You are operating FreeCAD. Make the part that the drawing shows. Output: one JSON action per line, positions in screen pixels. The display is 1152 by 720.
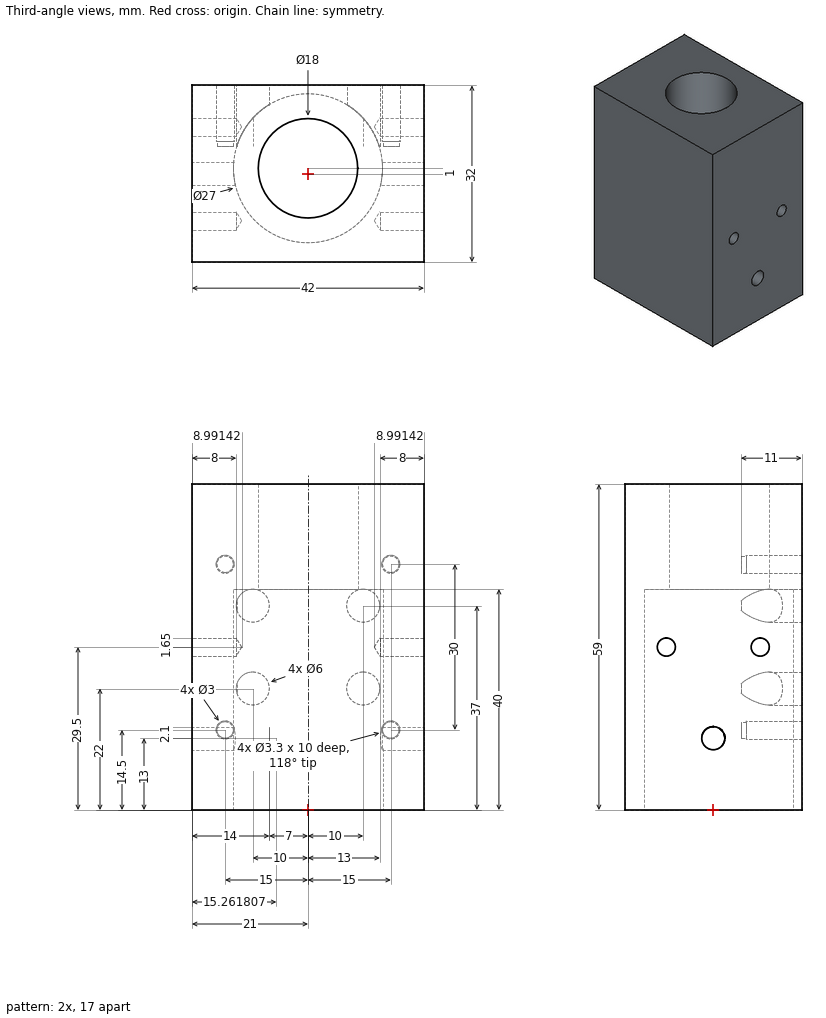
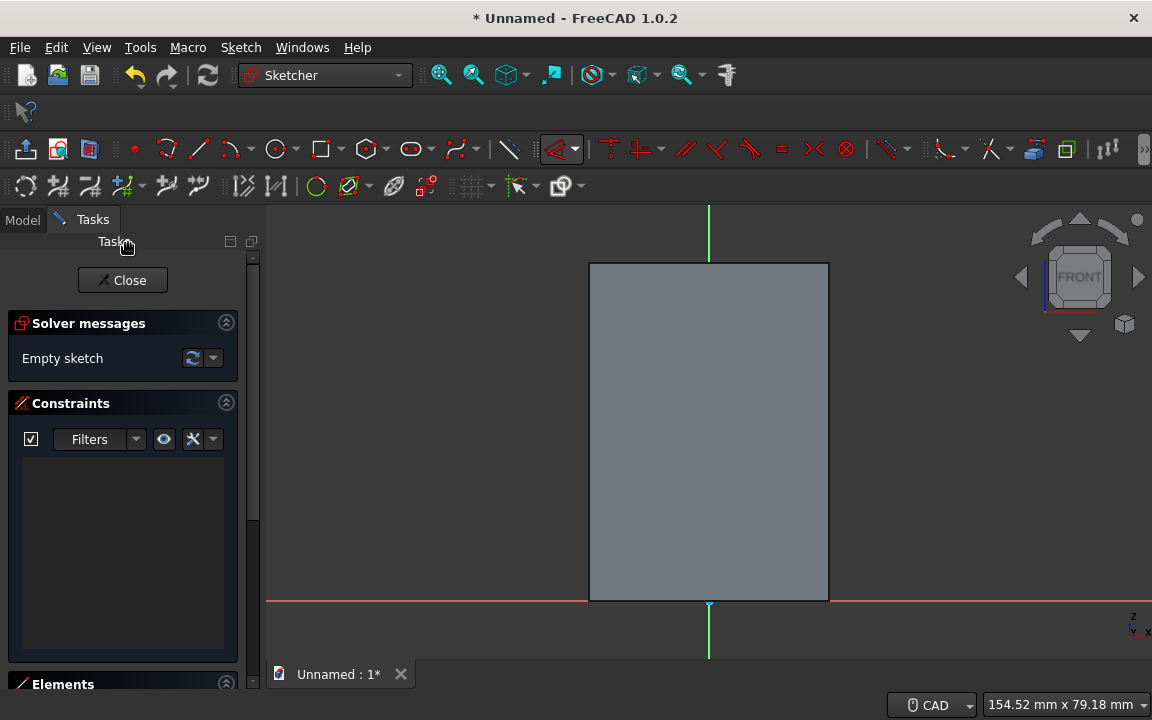
{"action": "key", "text": "q s"}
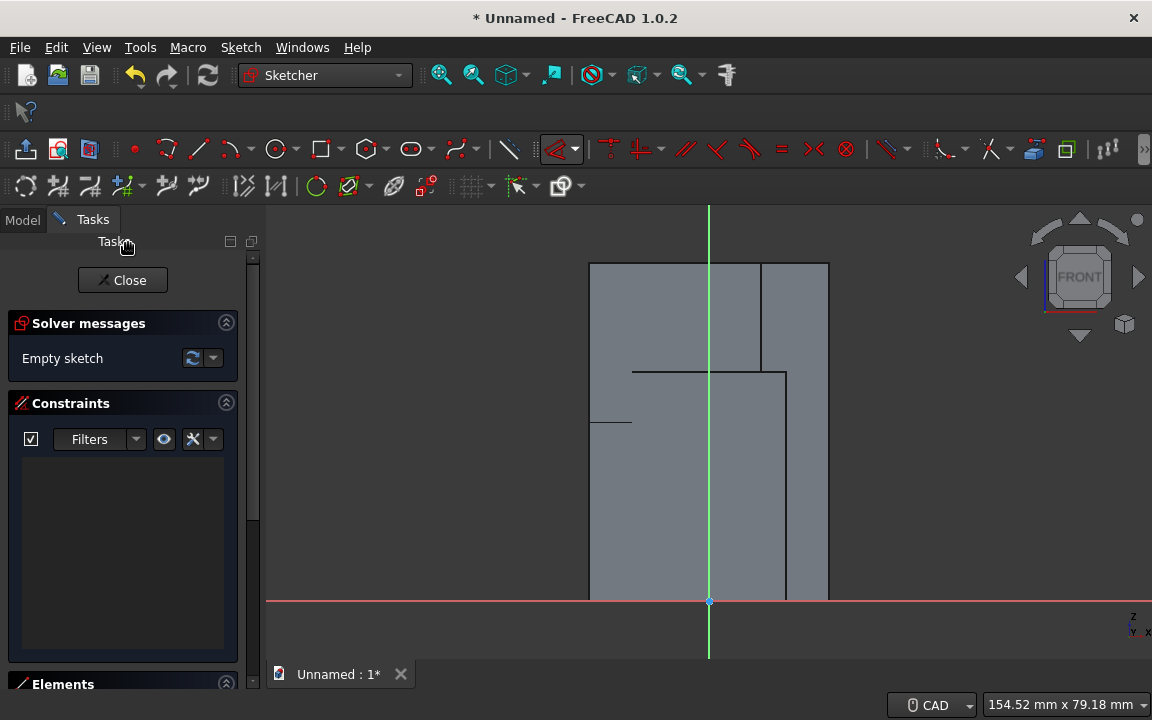
{"action": "scroll", "coordinate": [654, 612], "scroll_direction": "up", "scroll_amount": 6}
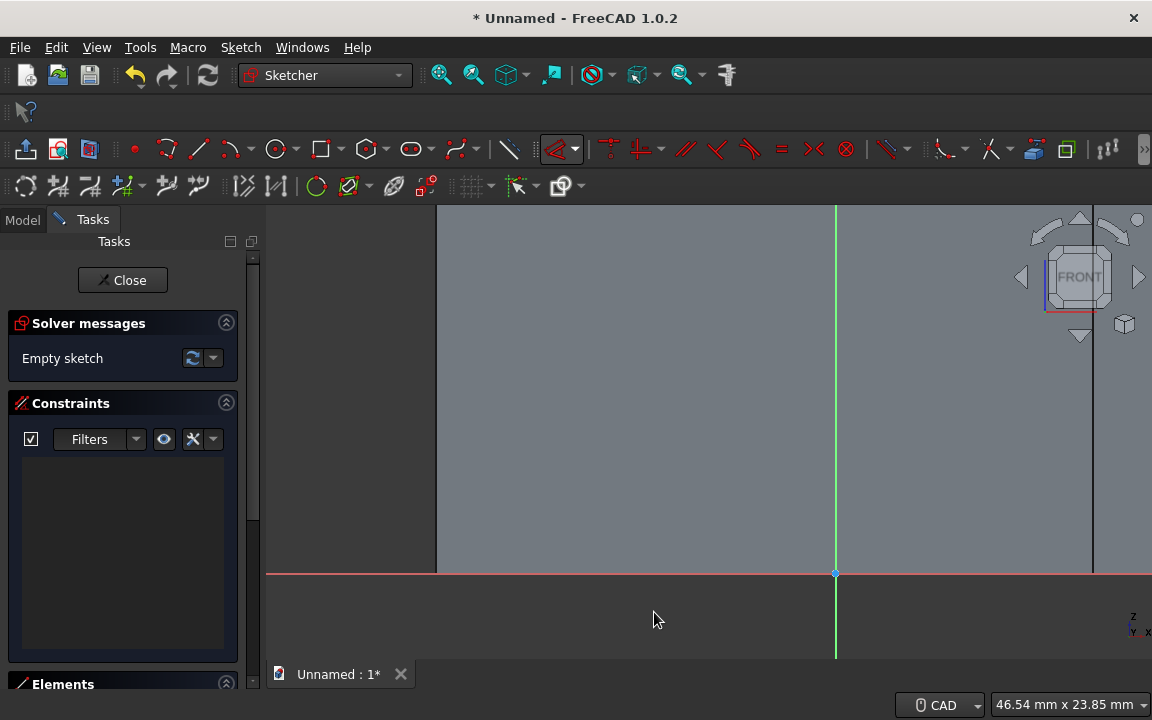
{"action": "left_click", "coordinate": [168, 150]}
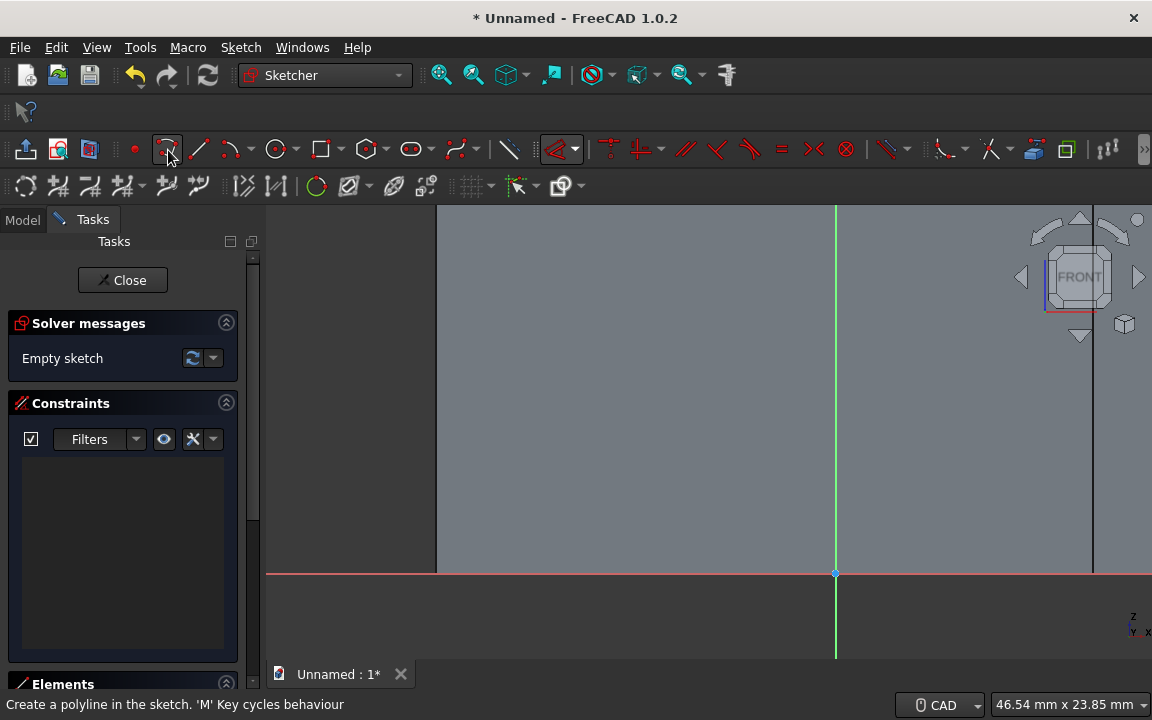
{"action": "left_click", "coordinate": [726, 326]}
{"action": "left_click", "coordinate": [436, 326]}
{"action": "left_click", "coordinate": [436, 286]}
{"action": "left_click", "coordinate": [702, 286]}
{"action": "left_click", "coordinate": [726, 327]}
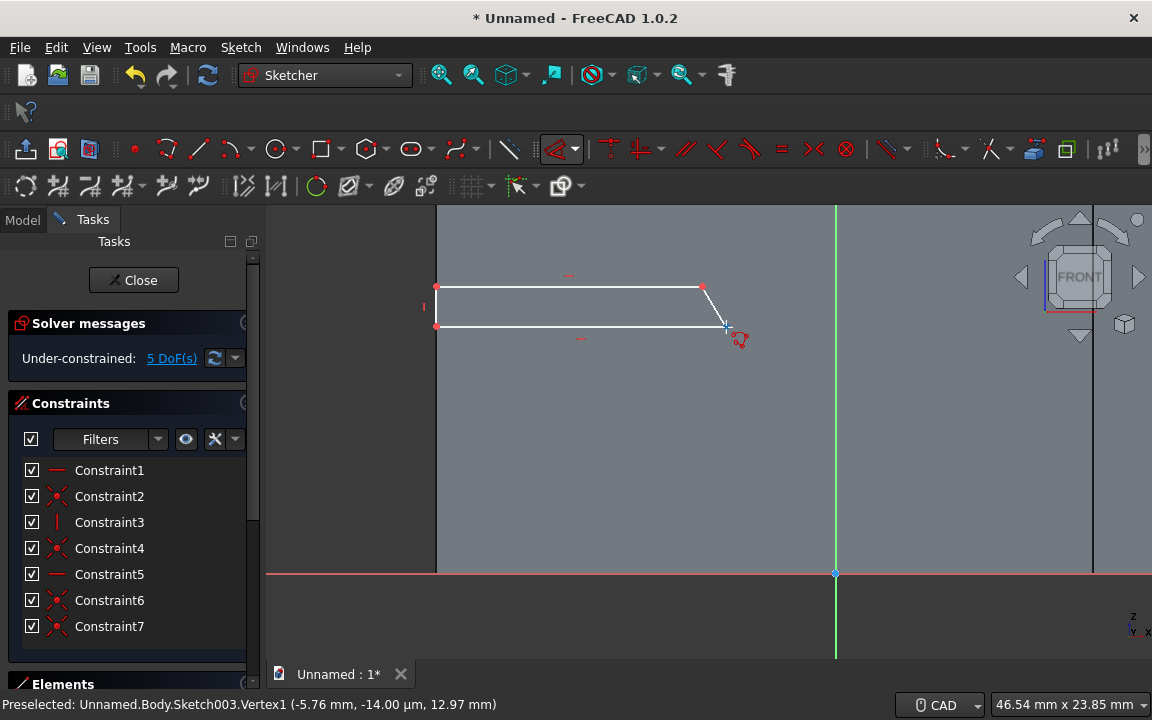
{"action": "key", "text": "g l"}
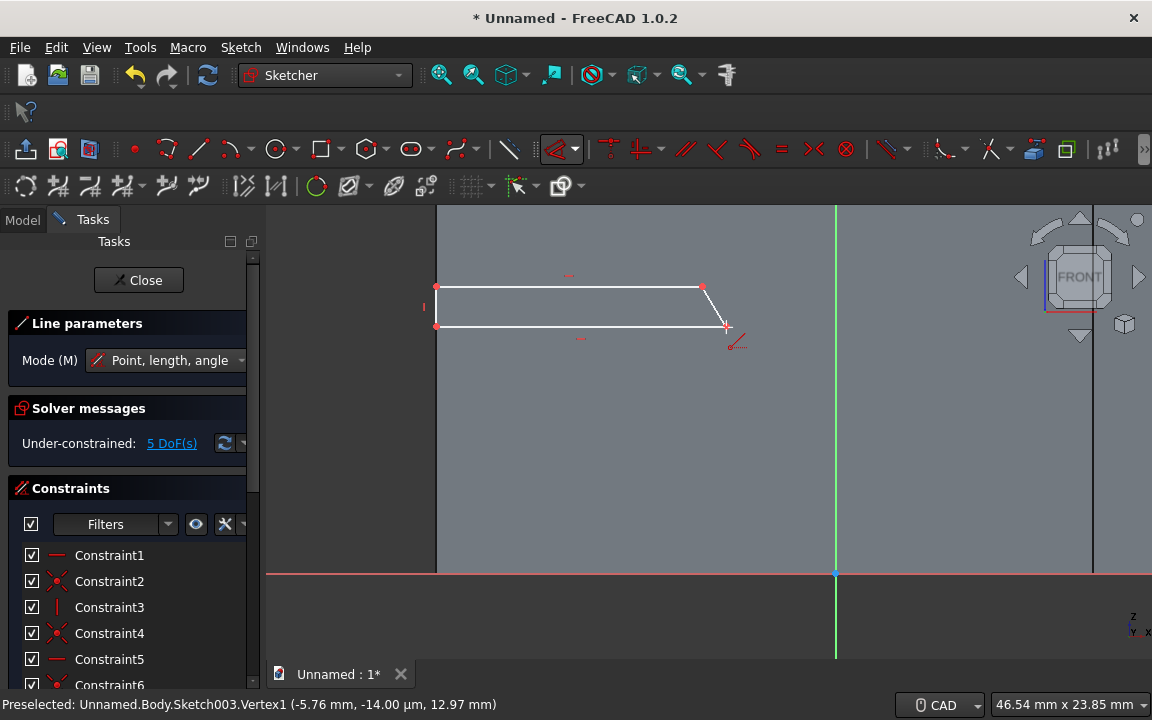
{"action": "left_click", "coordinate": [755, 326]}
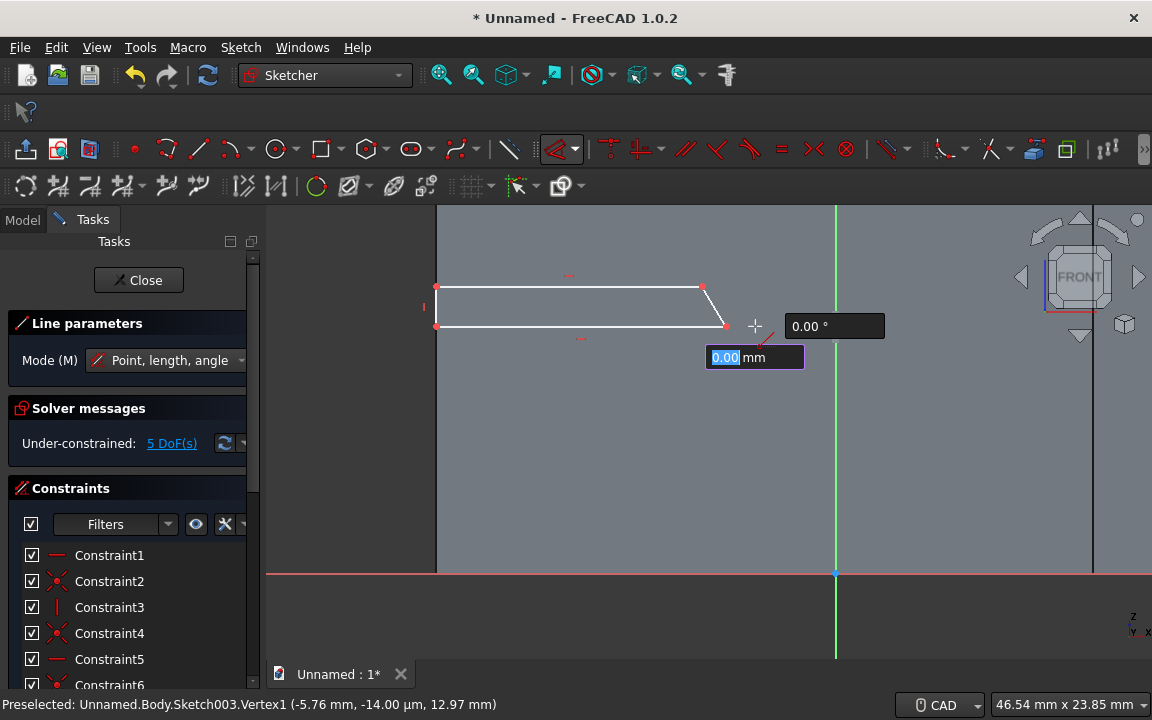
{"action": "scroll", "coordinate": [843, 326], "scroll_direction": "up", "scroll_amount": 5}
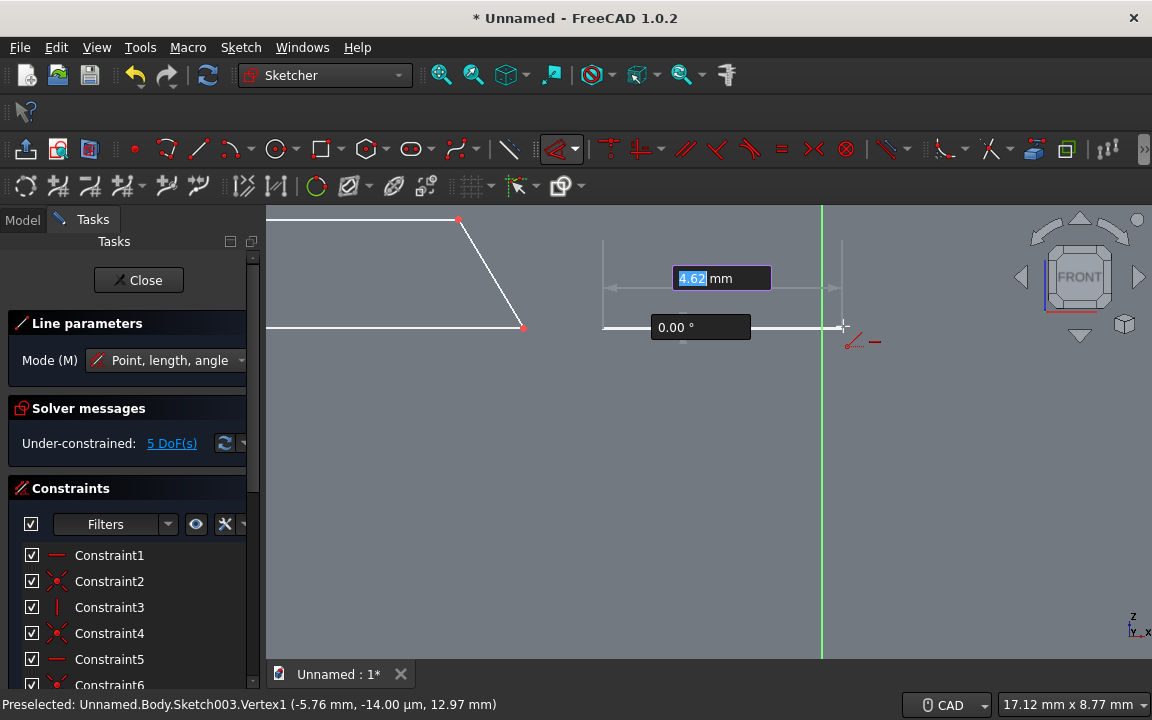
{"action": "left_click", "coordinate": [841, 326]}
{"action": "key", "text": "Escape"}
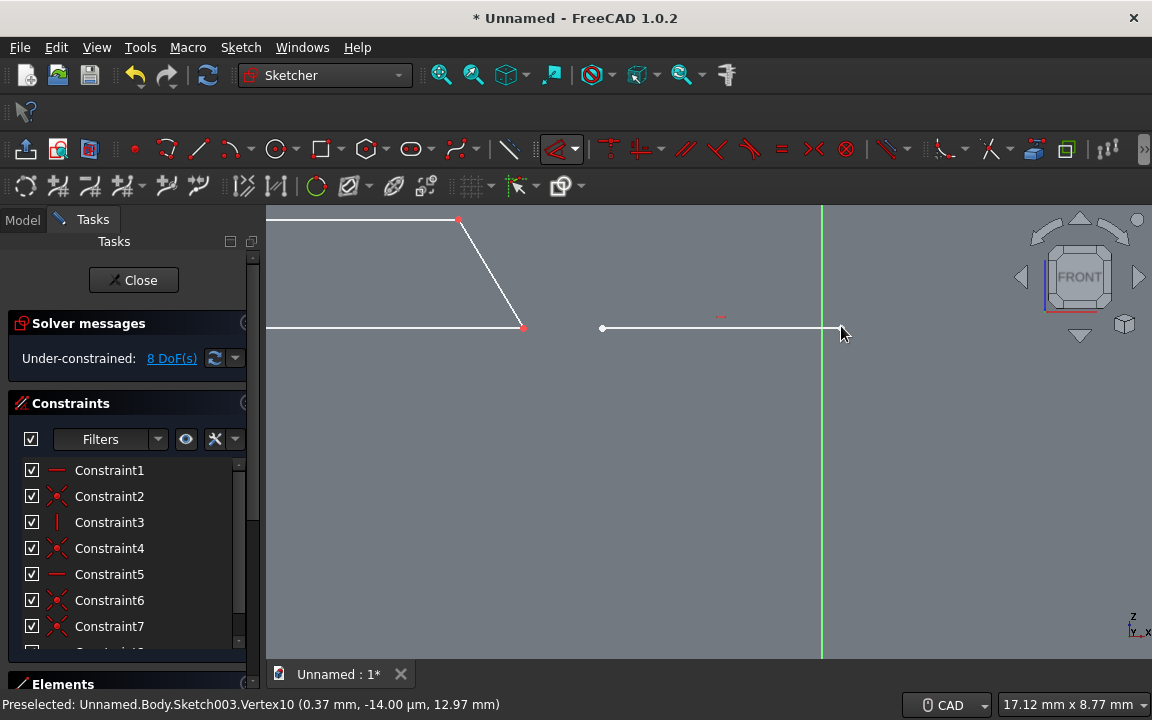
{"action": "left_click", "coordinate": [674, 328]}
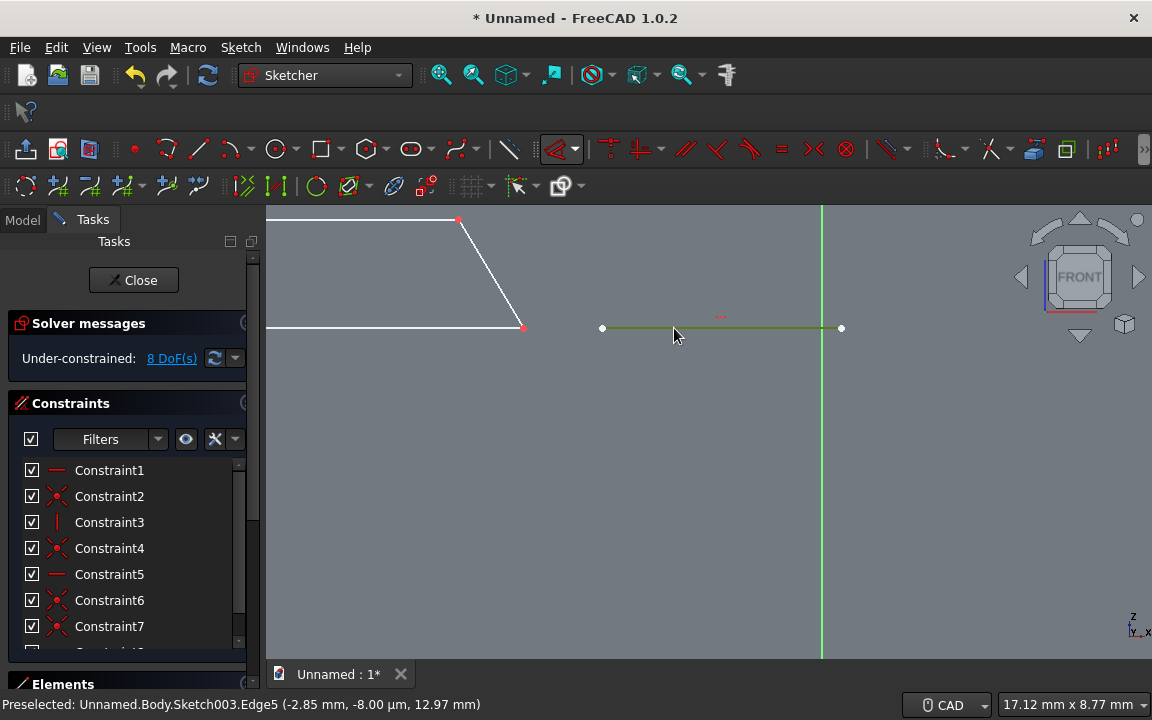
{"action": "left_click", "coordinate": [510, 150]}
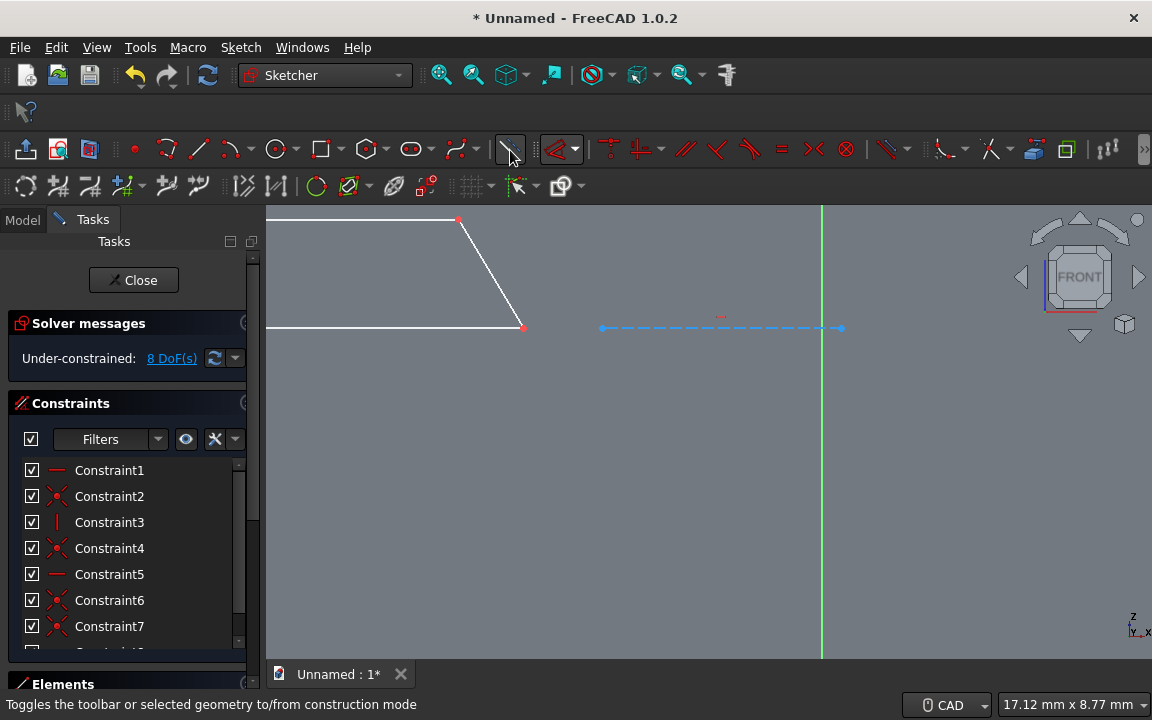
{"action": "scroll", "coordinate": [846, 329], "scroll_direction": "down", "scroll_amount": 5}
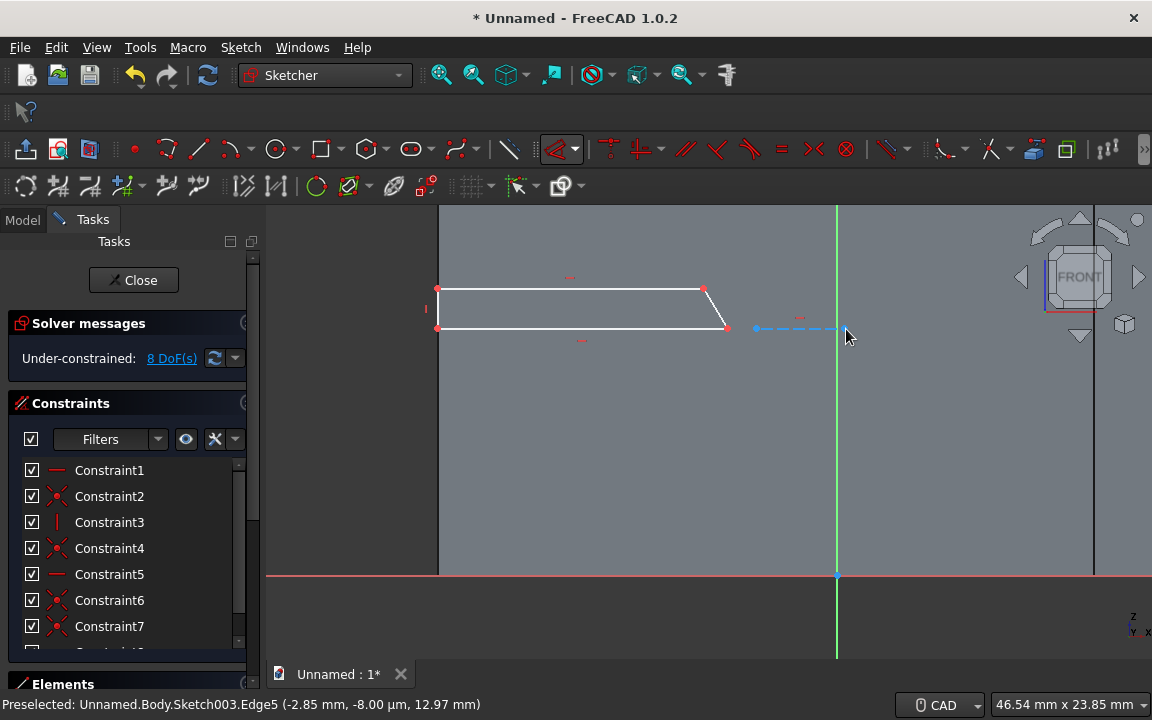
{"action": "left_click", "coordinate": [518, 289]}